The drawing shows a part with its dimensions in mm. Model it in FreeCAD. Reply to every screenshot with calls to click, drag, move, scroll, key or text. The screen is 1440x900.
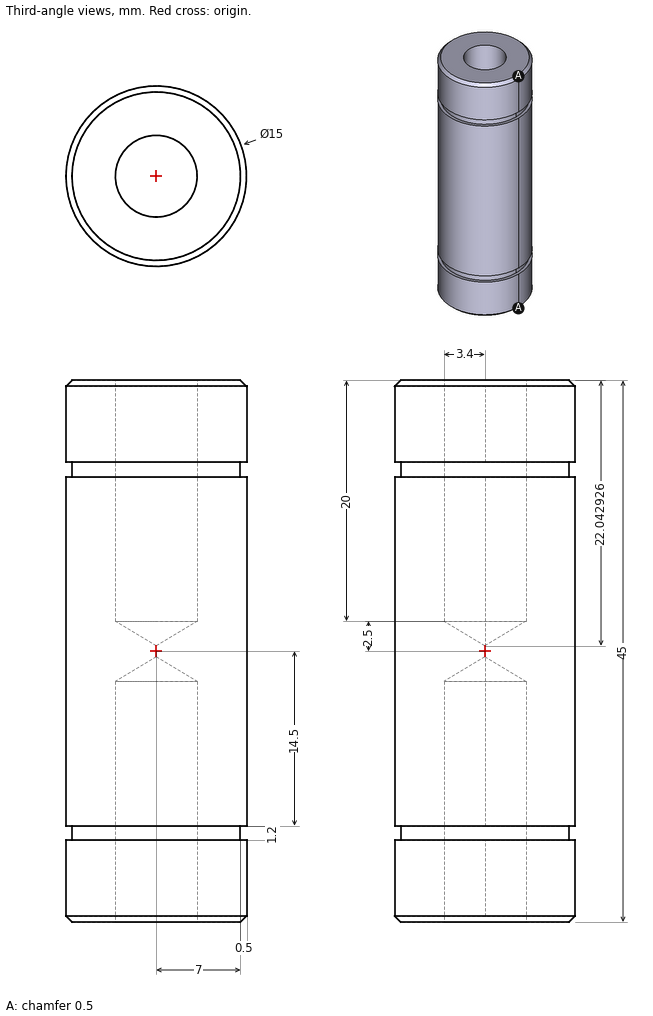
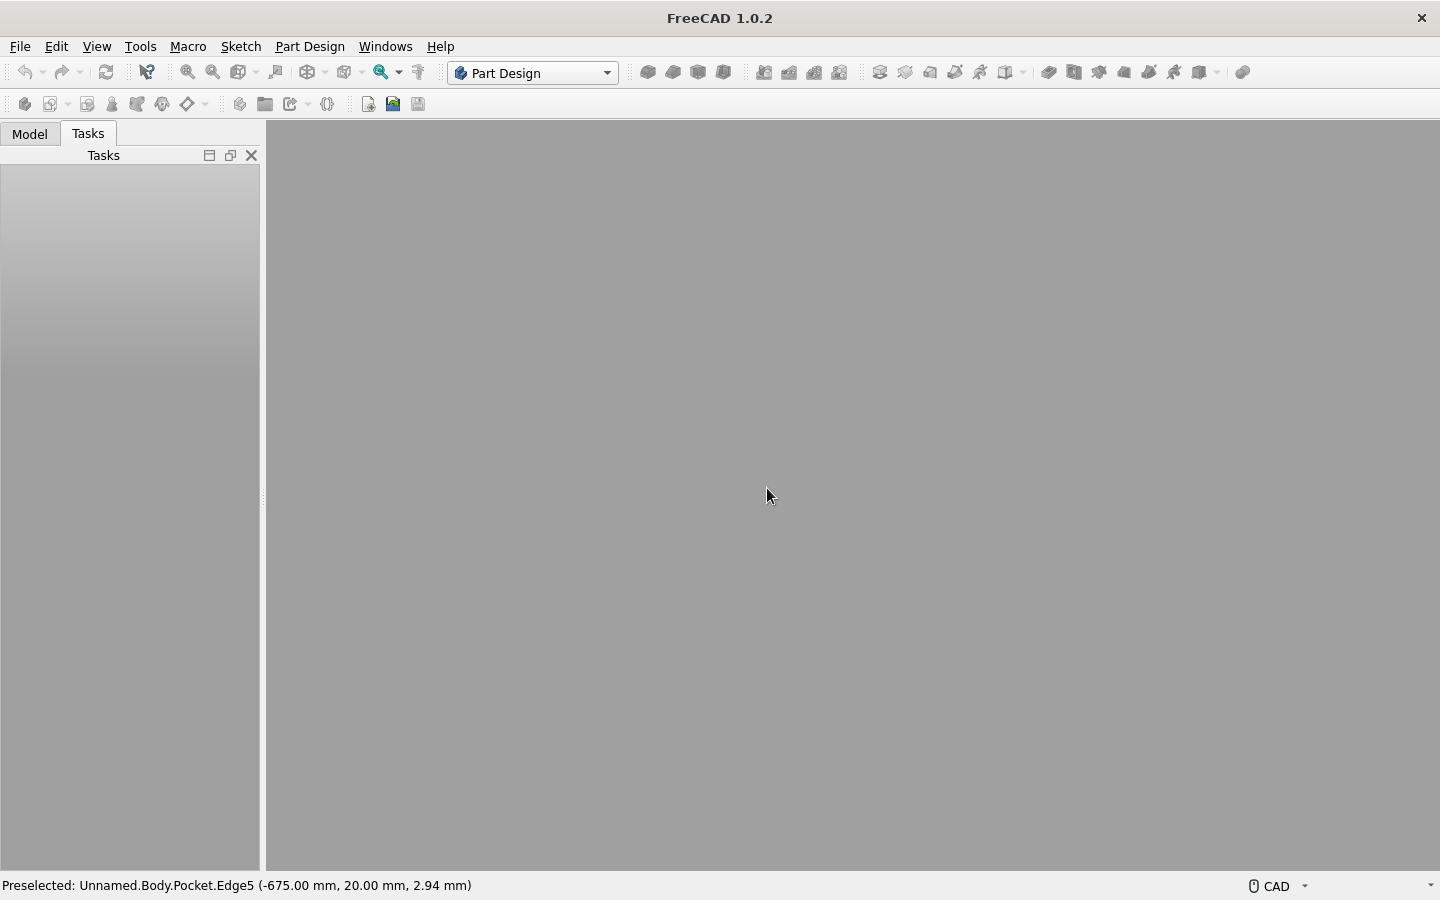
key(ctrl+n)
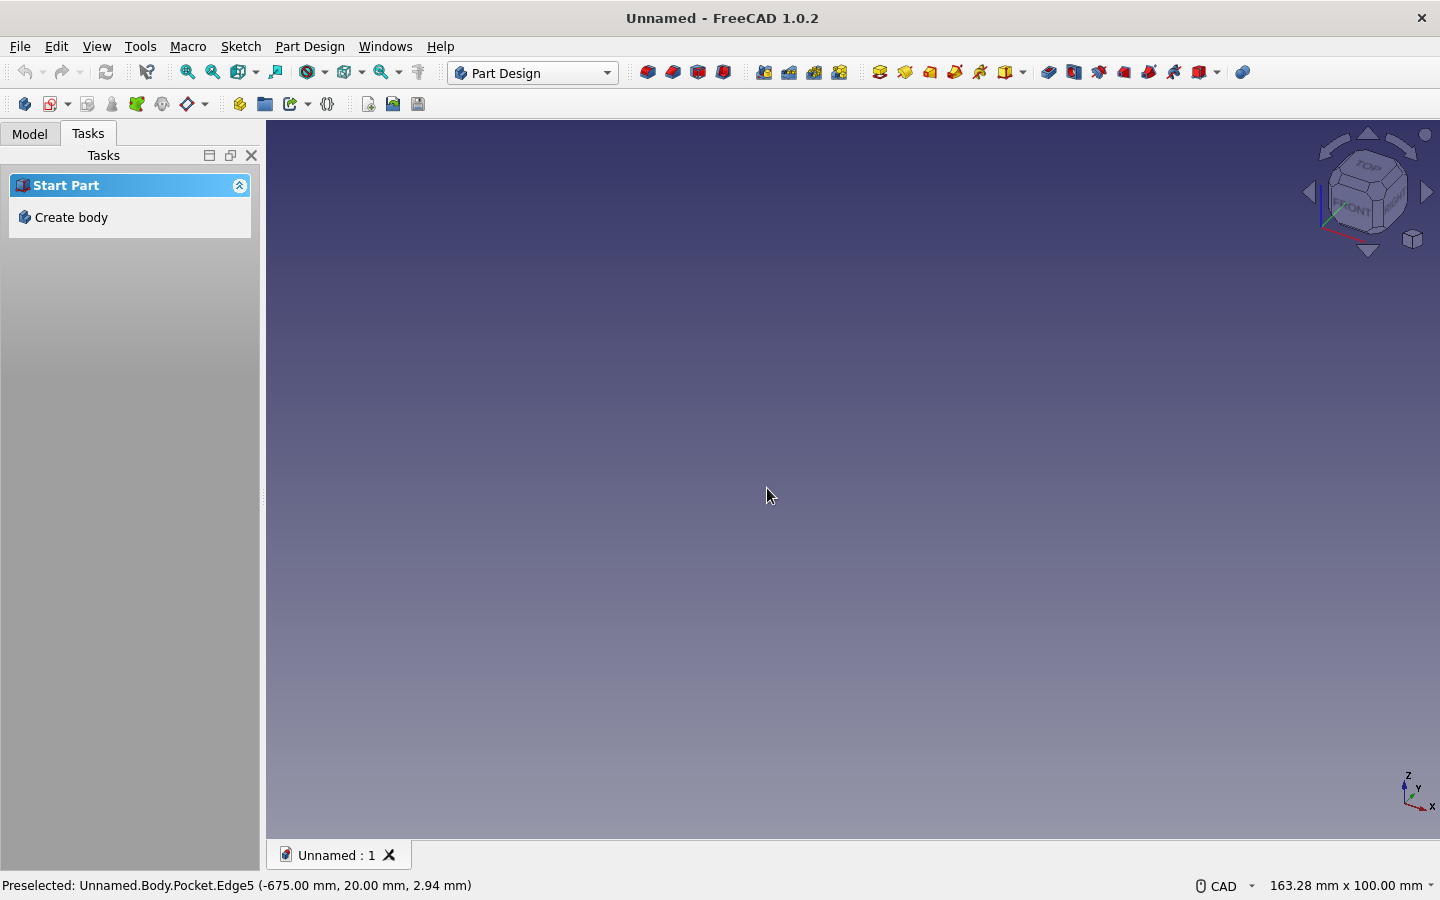
click(50, 104)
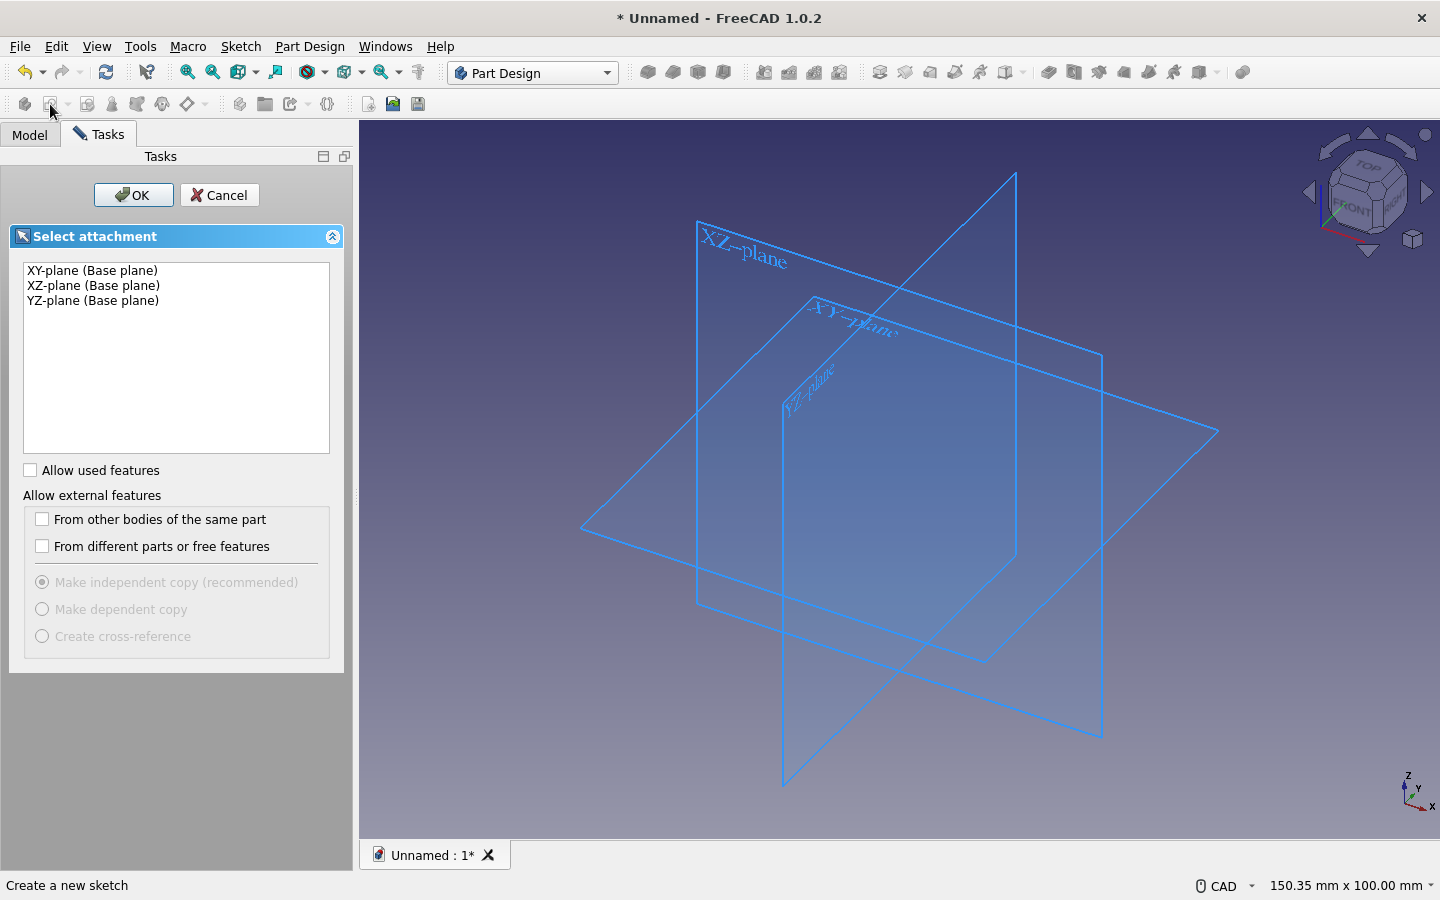
click(84, 270)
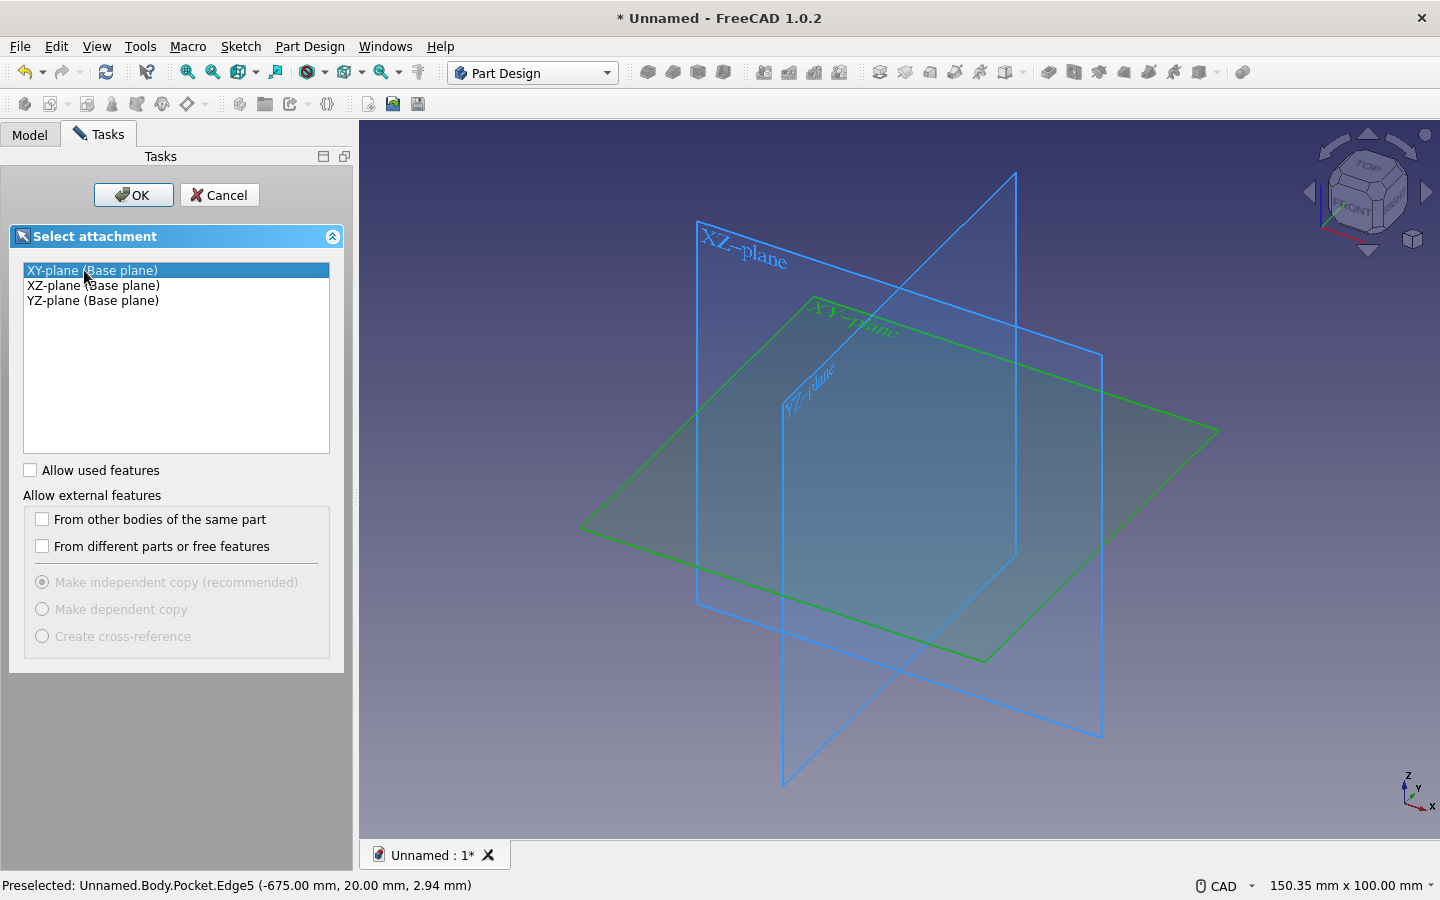
click(134, 195)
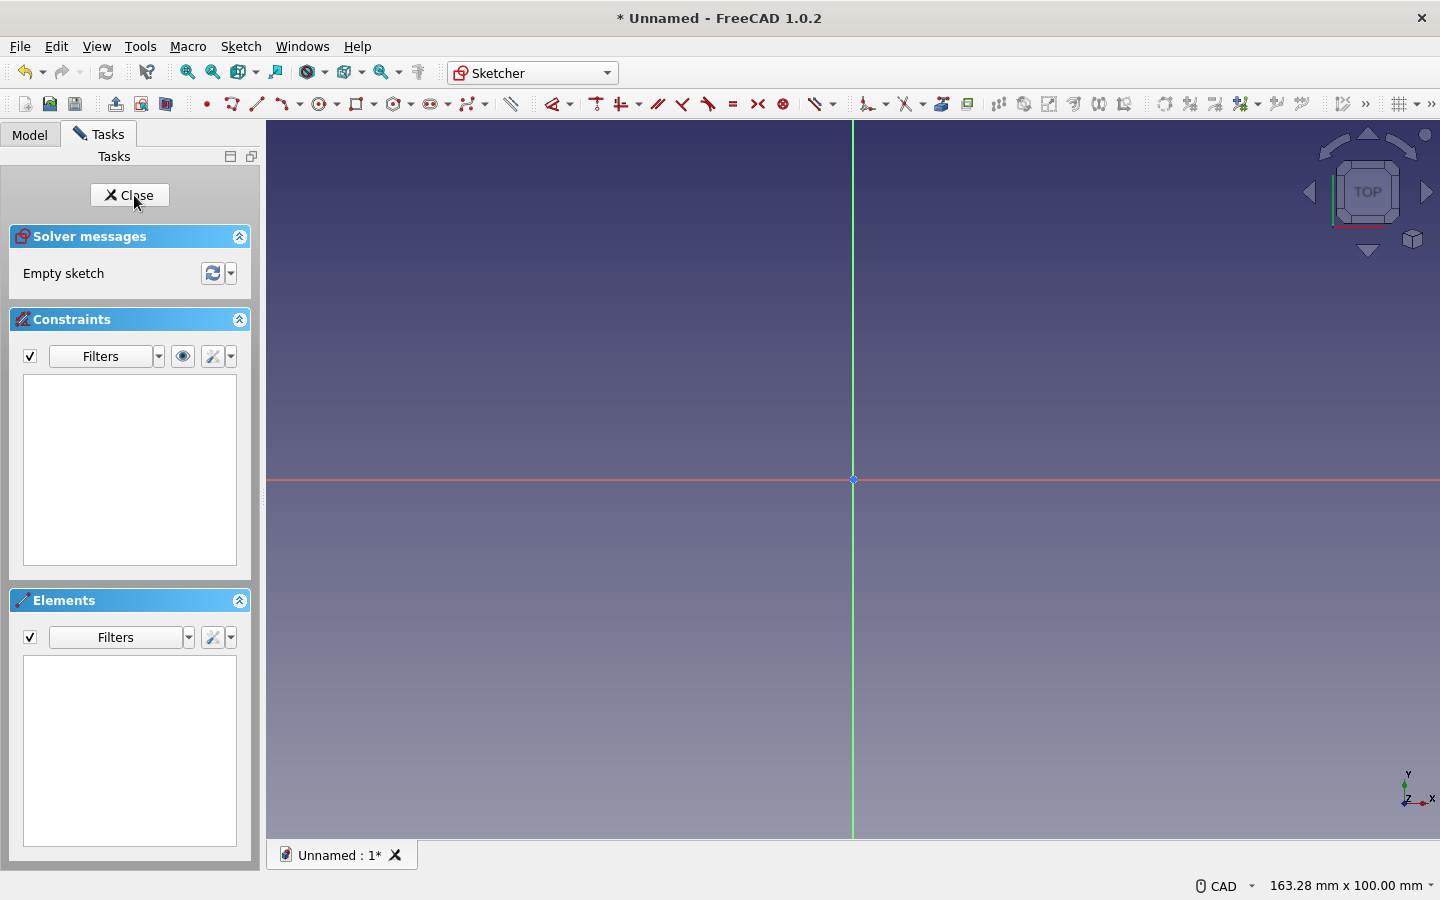
scroll(875, 480, up, 7)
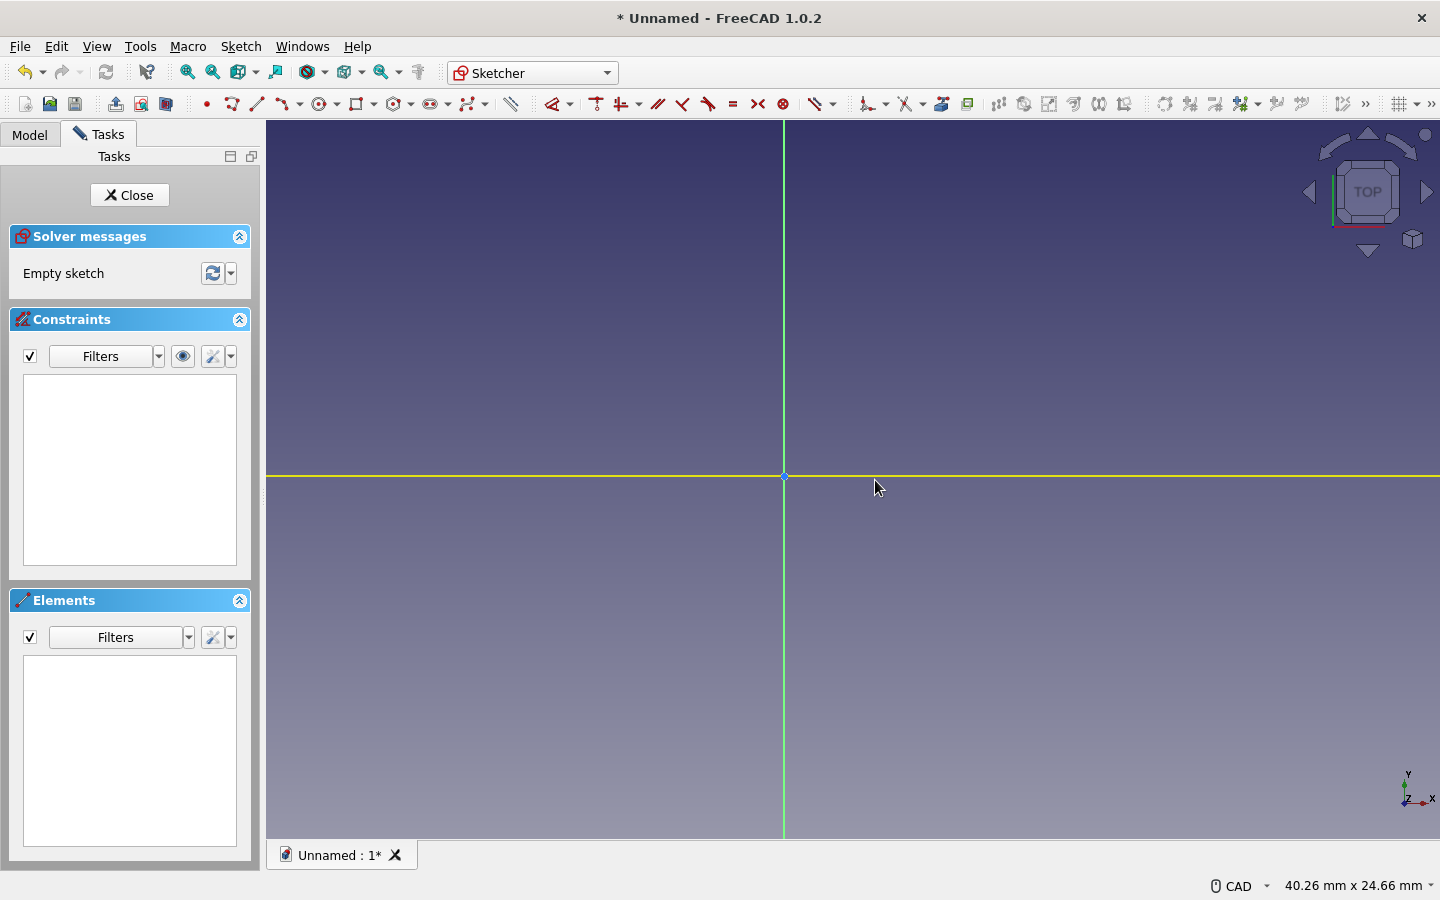
click(318, 104)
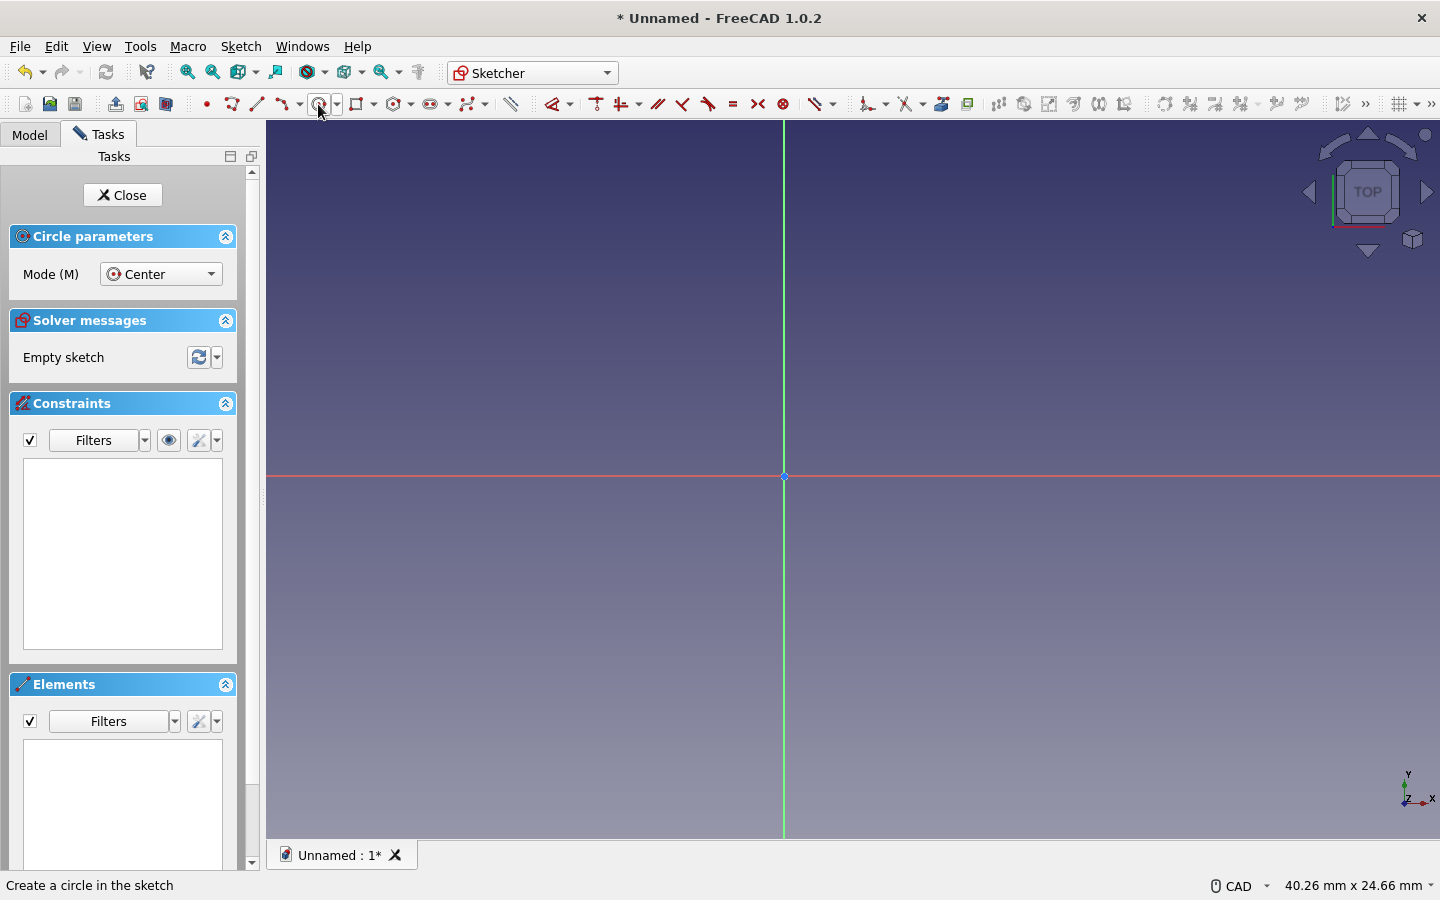
click(784, 476)
click(939, 322)
key(Escape)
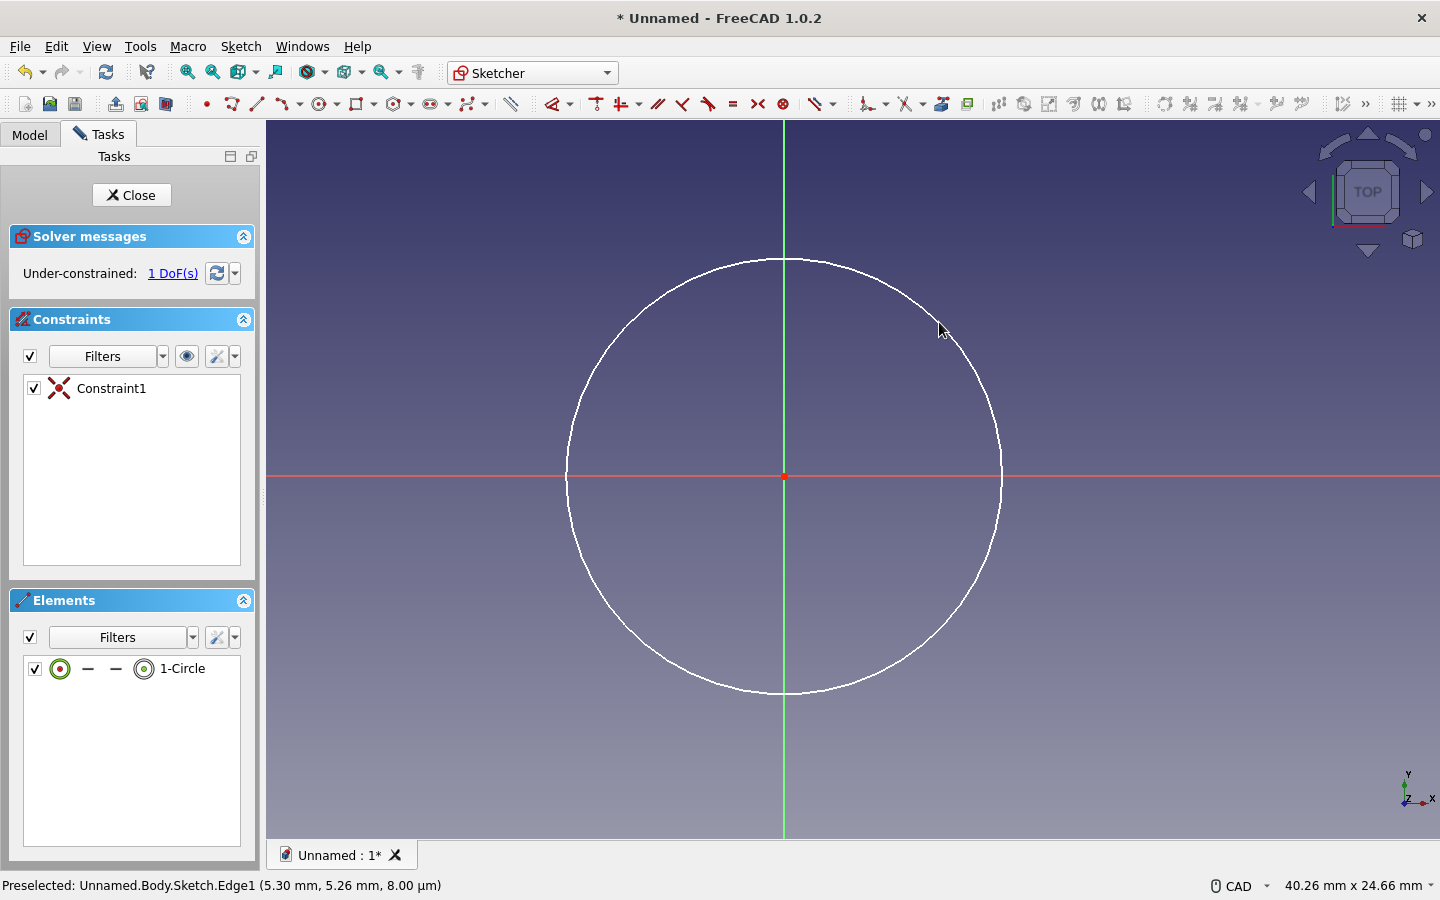
click(938, 322)